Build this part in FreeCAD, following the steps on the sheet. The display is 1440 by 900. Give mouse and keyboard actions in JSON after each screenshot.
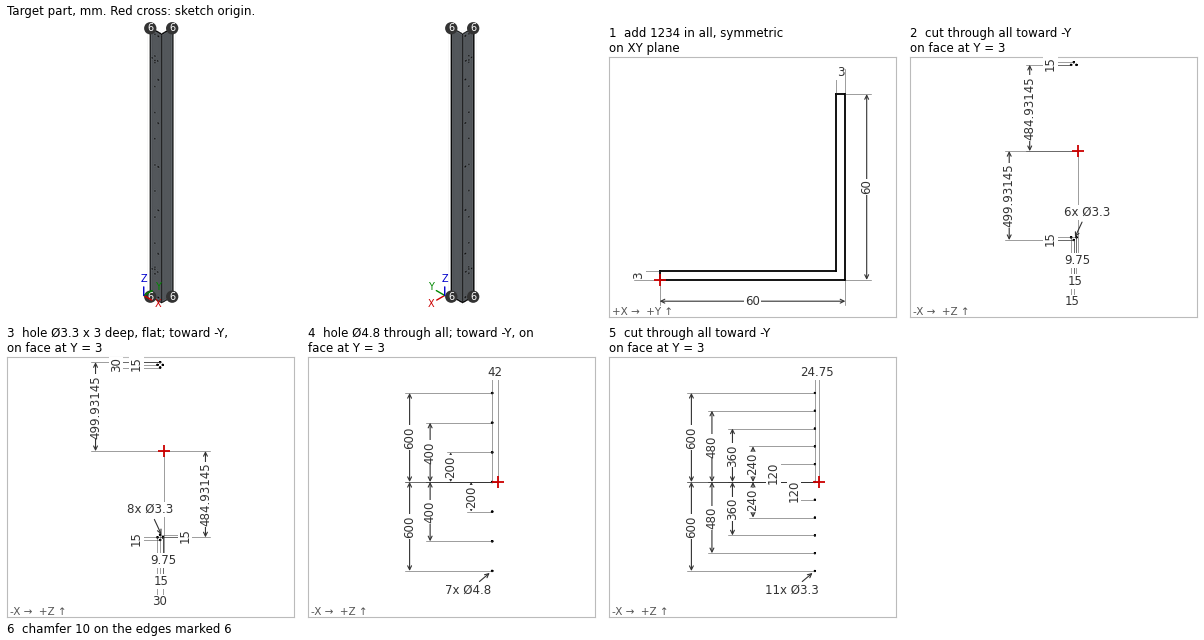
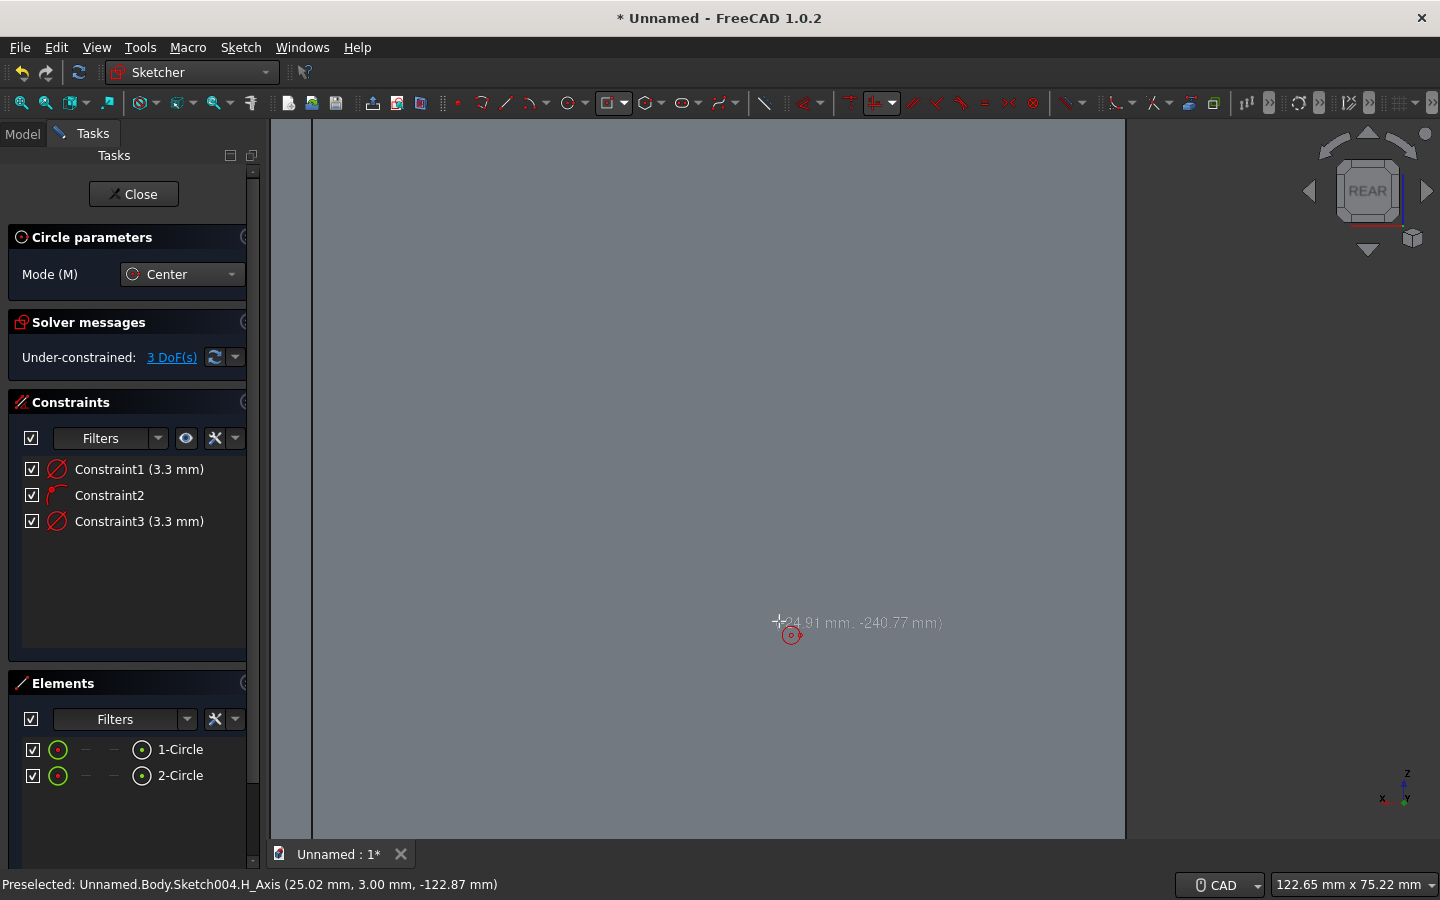
{"action": "scroll", "coordinate": [779, 593], "scroll_direction": "down", "scroll_amount": 17}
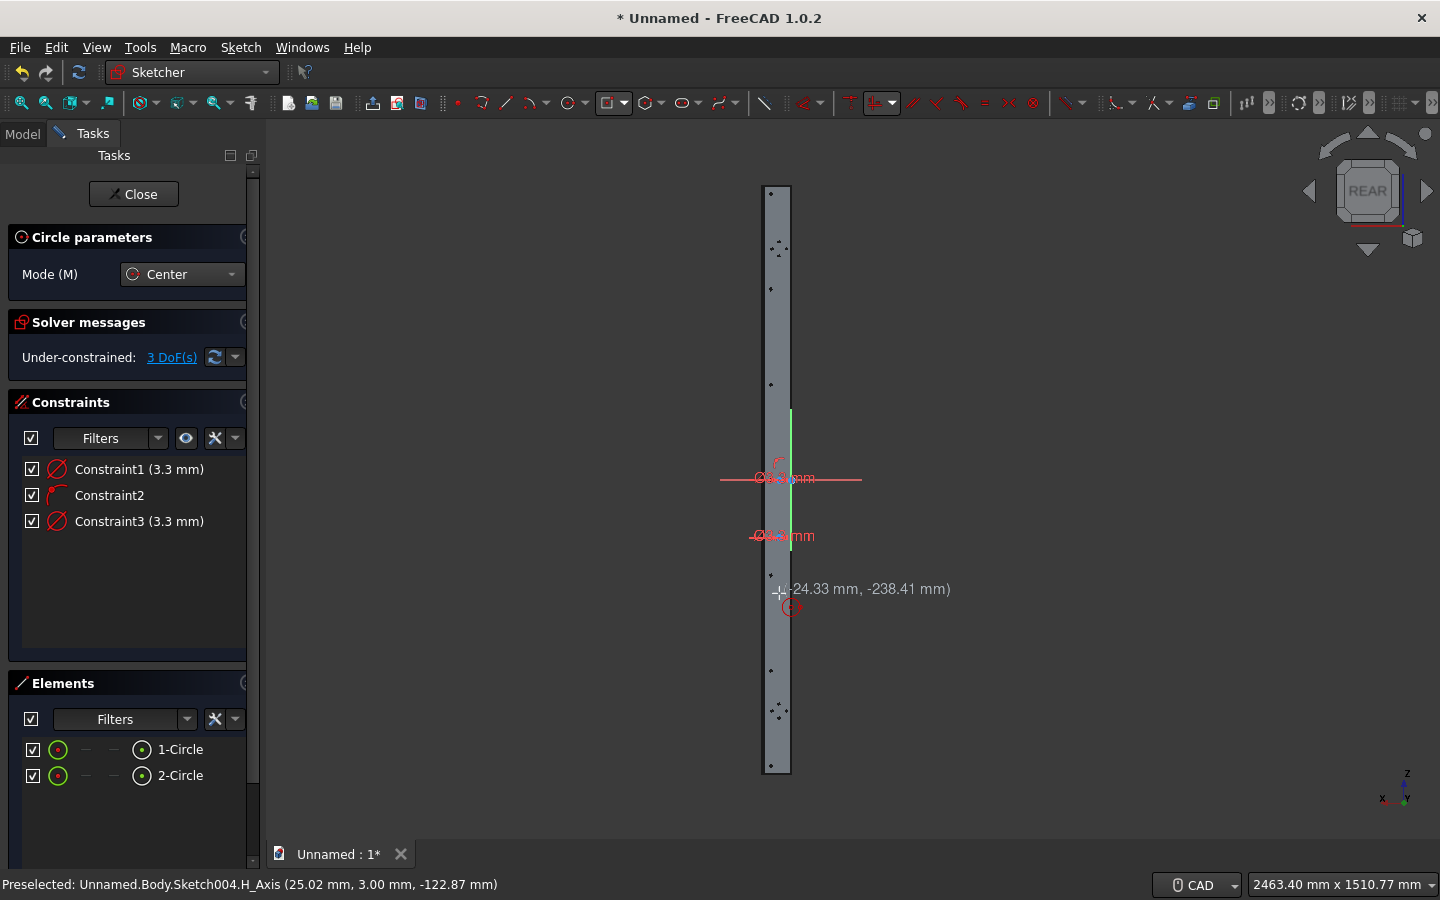
{"action": "scroll", "coordinate": [779, 594], "scroll_direction": "up", "scroll_amount": 2}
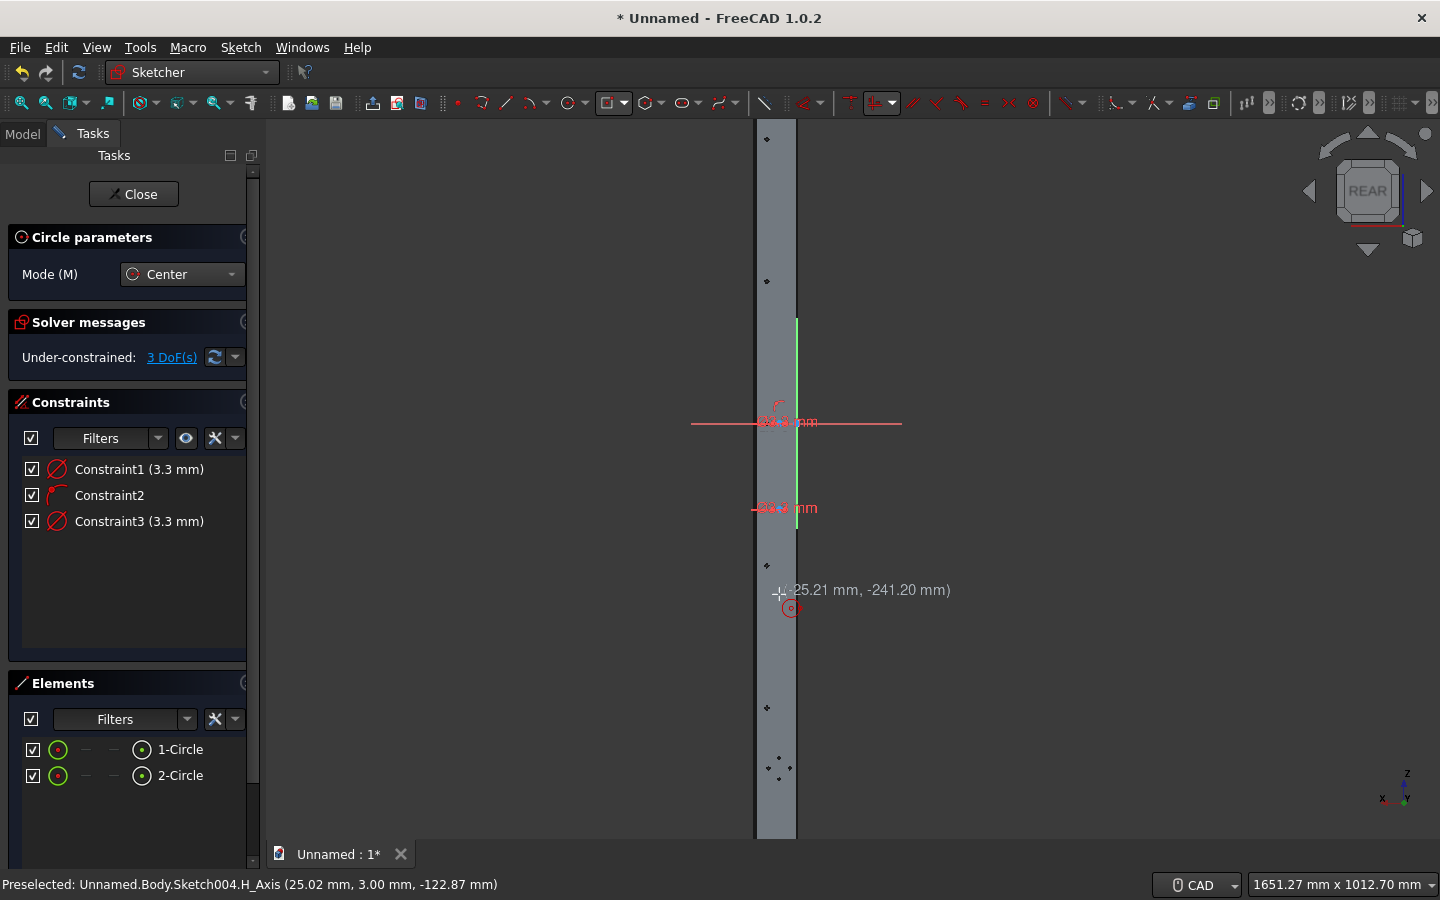
{"action": "left_click", "coordinate": [779, 594]}
{"action": "mouse_move", "coordinate": [780, 593]}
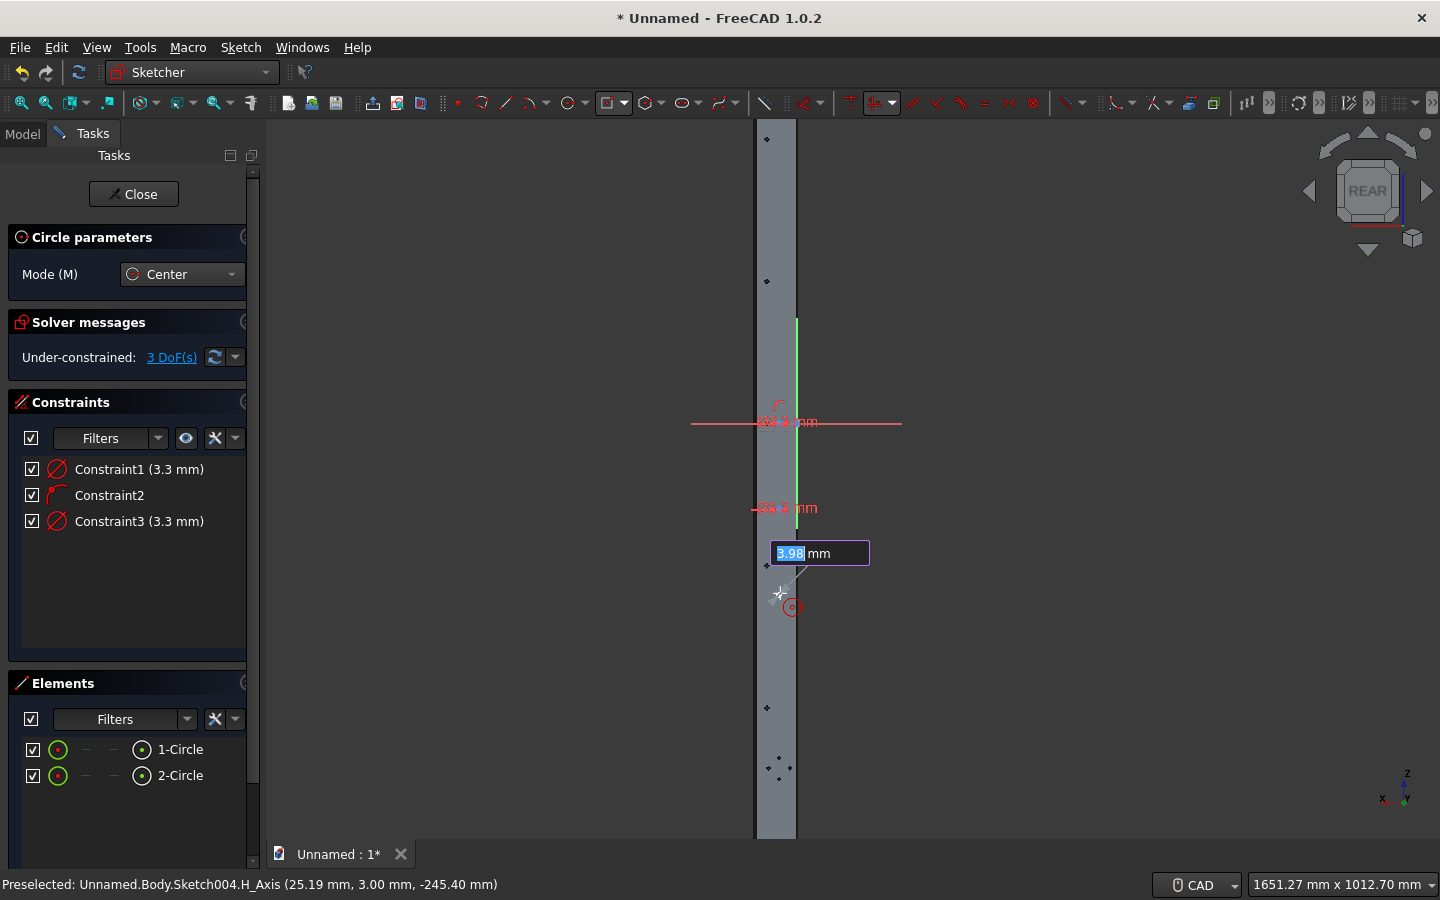
{"action": "type", "text": "3.3"}
{"action": "key", "text": "Return"}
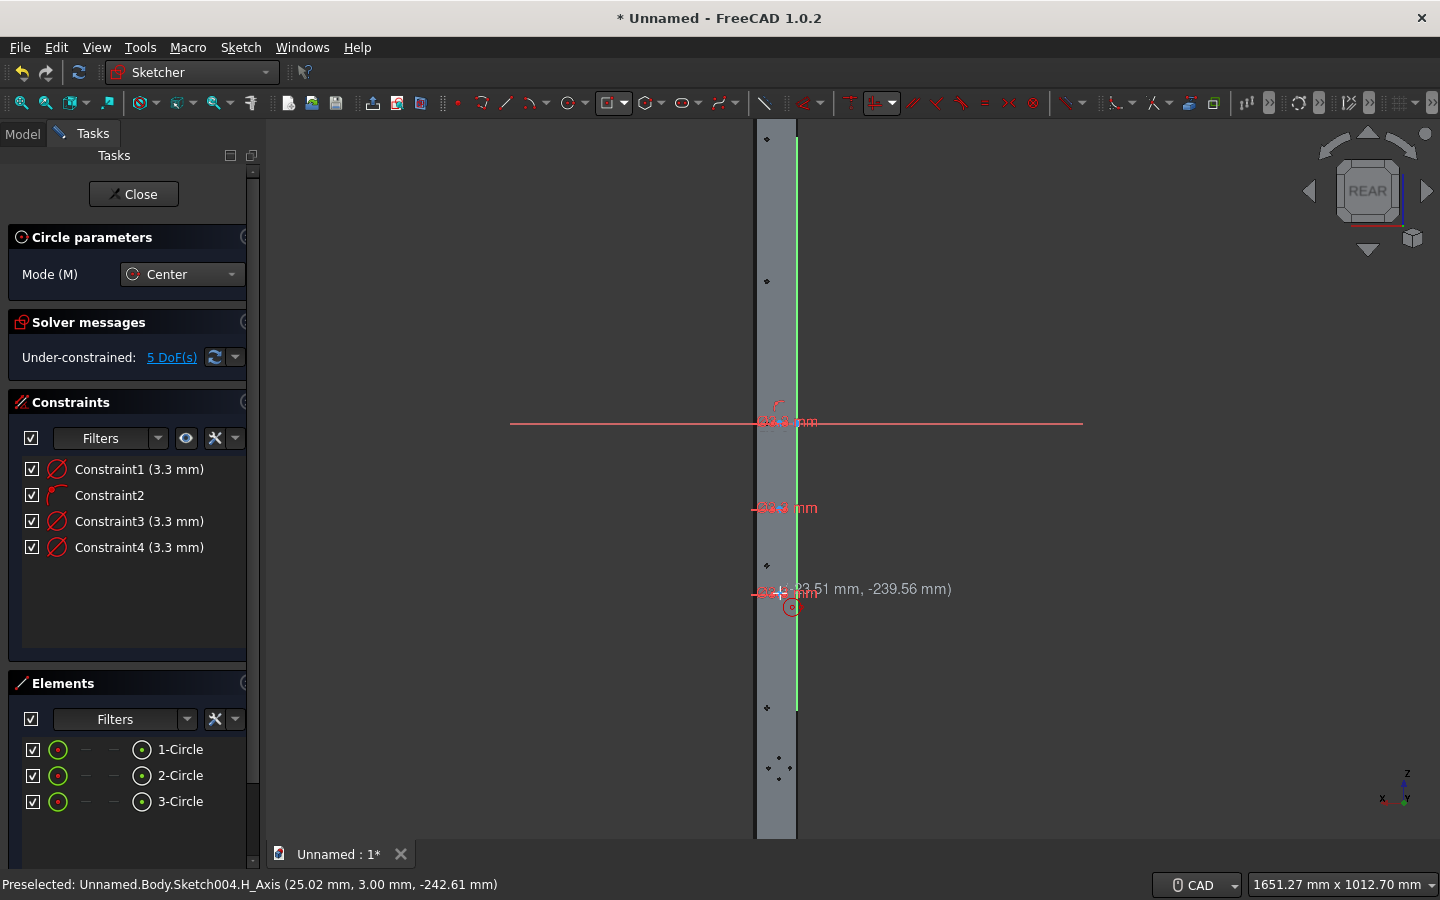
{"action": "scroll", "coordinate": [779, 680], "scroll_direction": "up", "scroll_amount": 15}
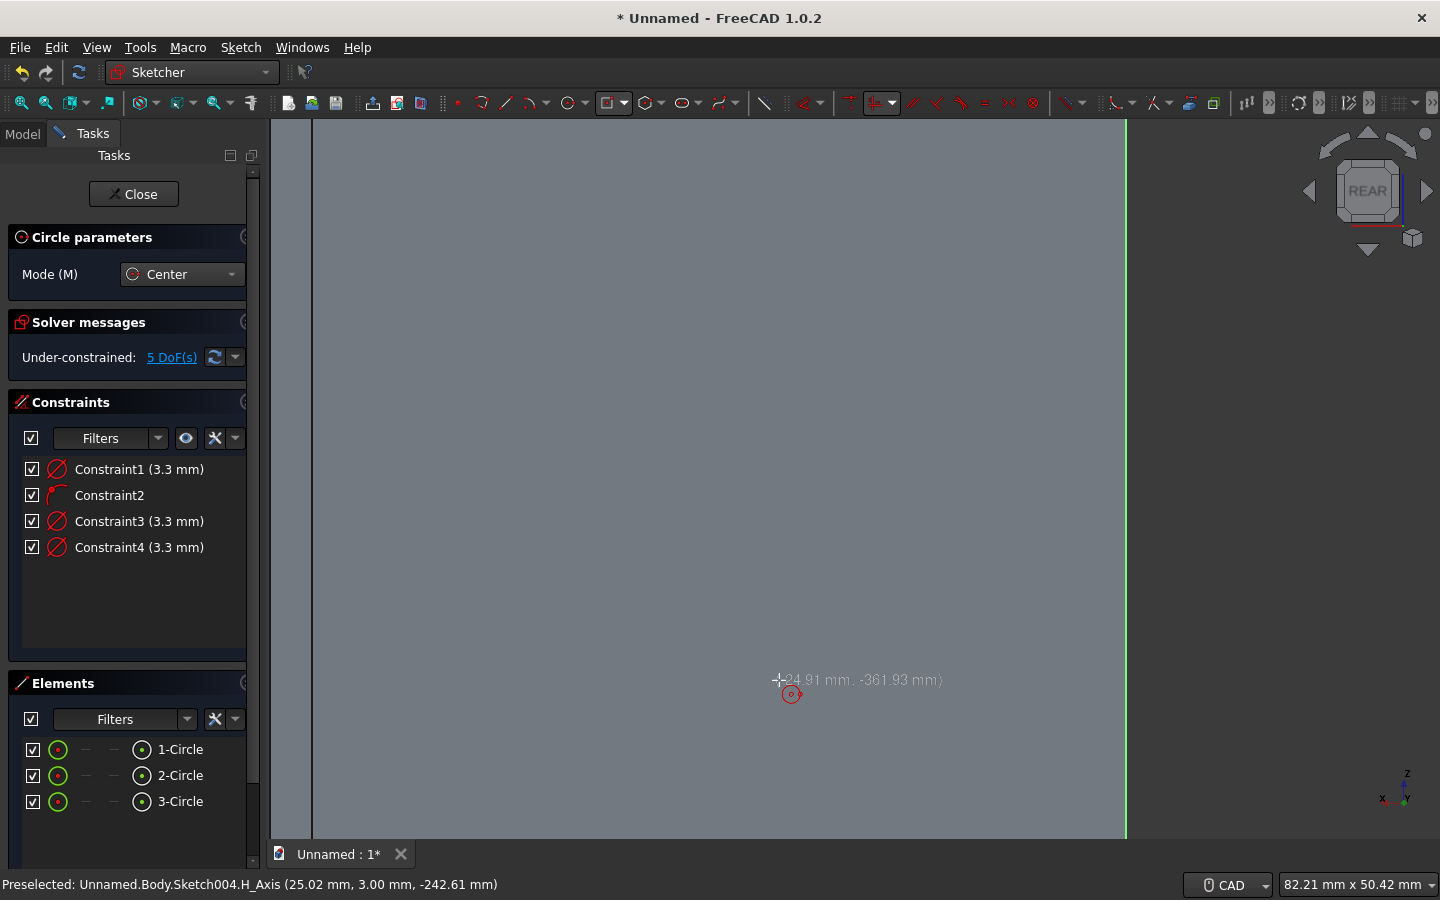
{"action": "scroll", "coordinate": [779, 650], "scroll_direction": "down", "scroll_amount": 17}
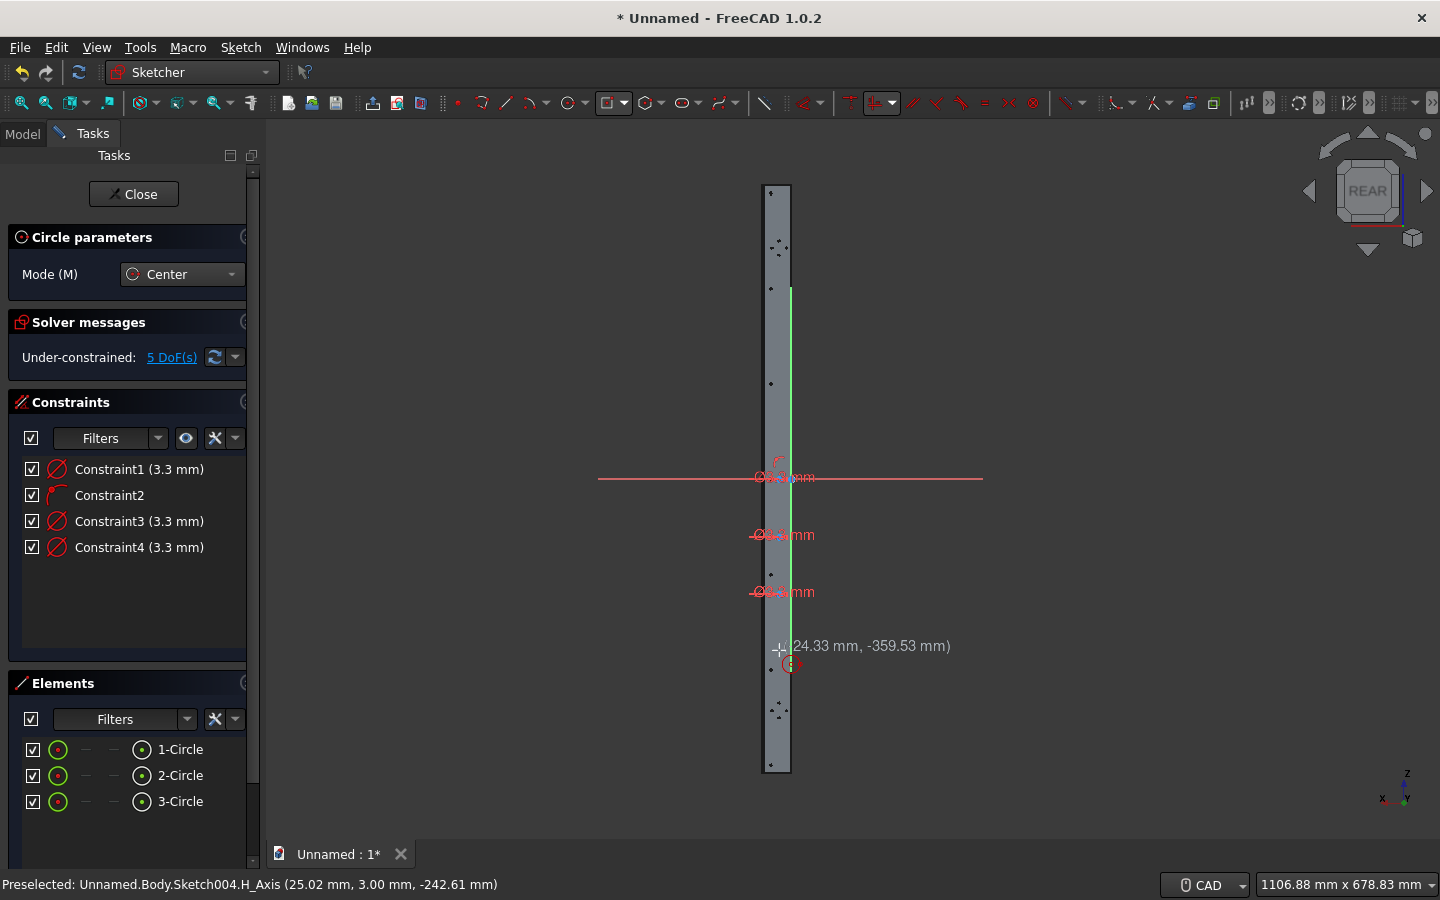
{"action": "scroll", "coordinate": [779, 651], "scroll_direction": "up", "scroll_amount": 2}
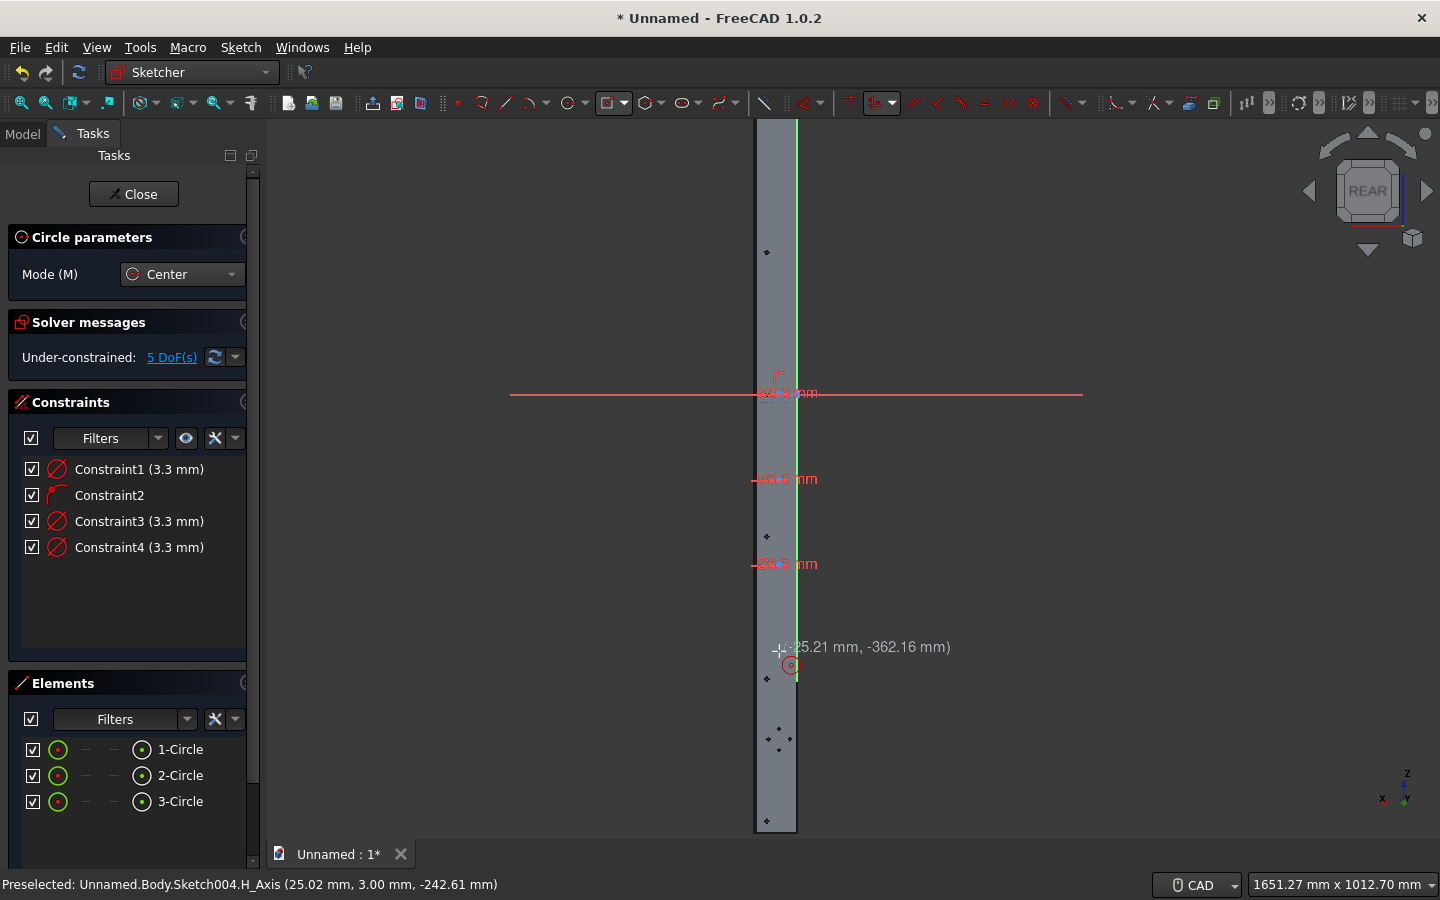
{"action": "left_click", "coordinate": [779, 651]}
{"action": "mouse_move", "coordinate": [780, 650]}